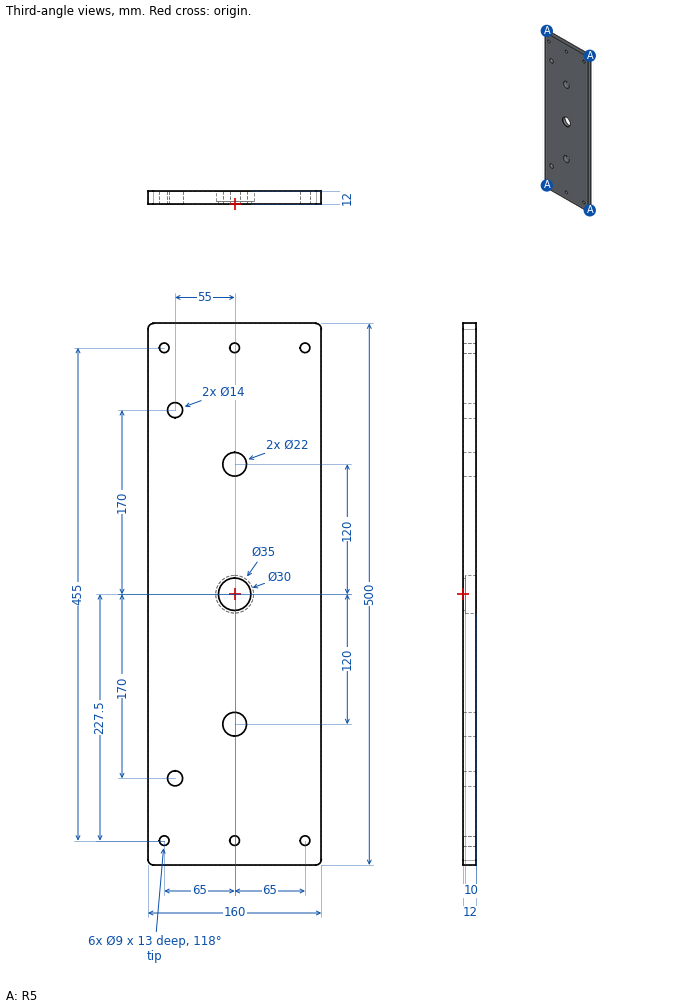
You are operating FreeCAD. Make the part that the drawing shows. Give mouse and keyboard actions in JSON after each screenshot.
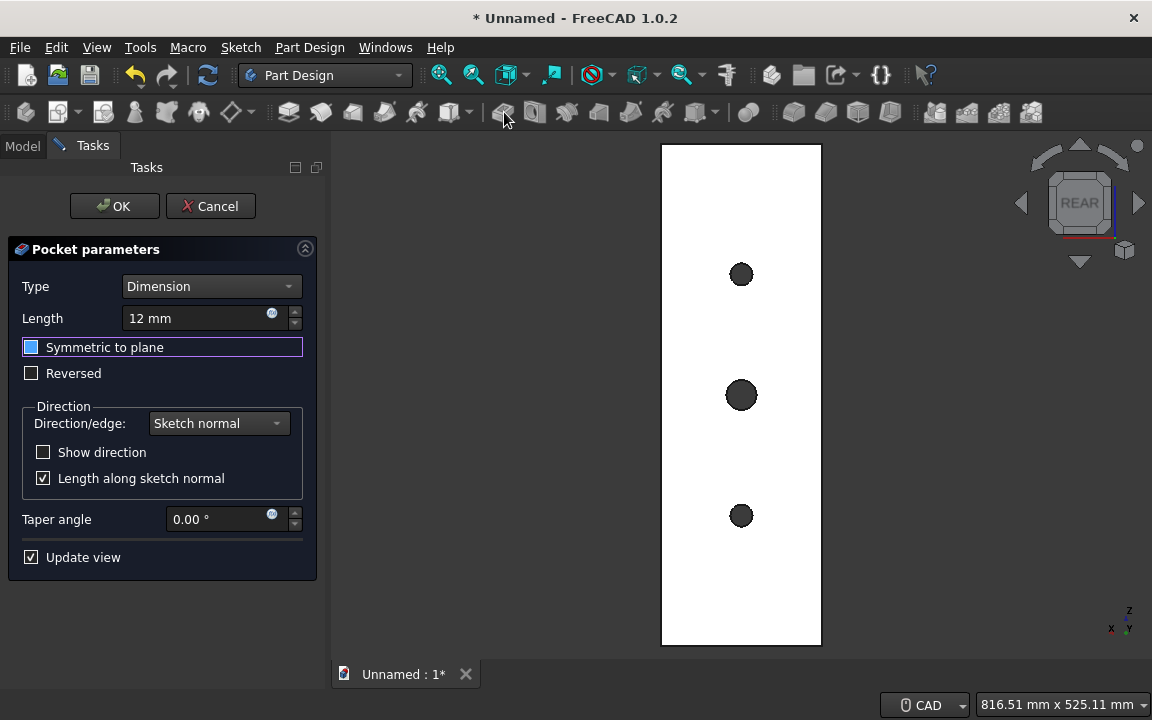
{"action": "left_click", "coordinate": [115, 206]}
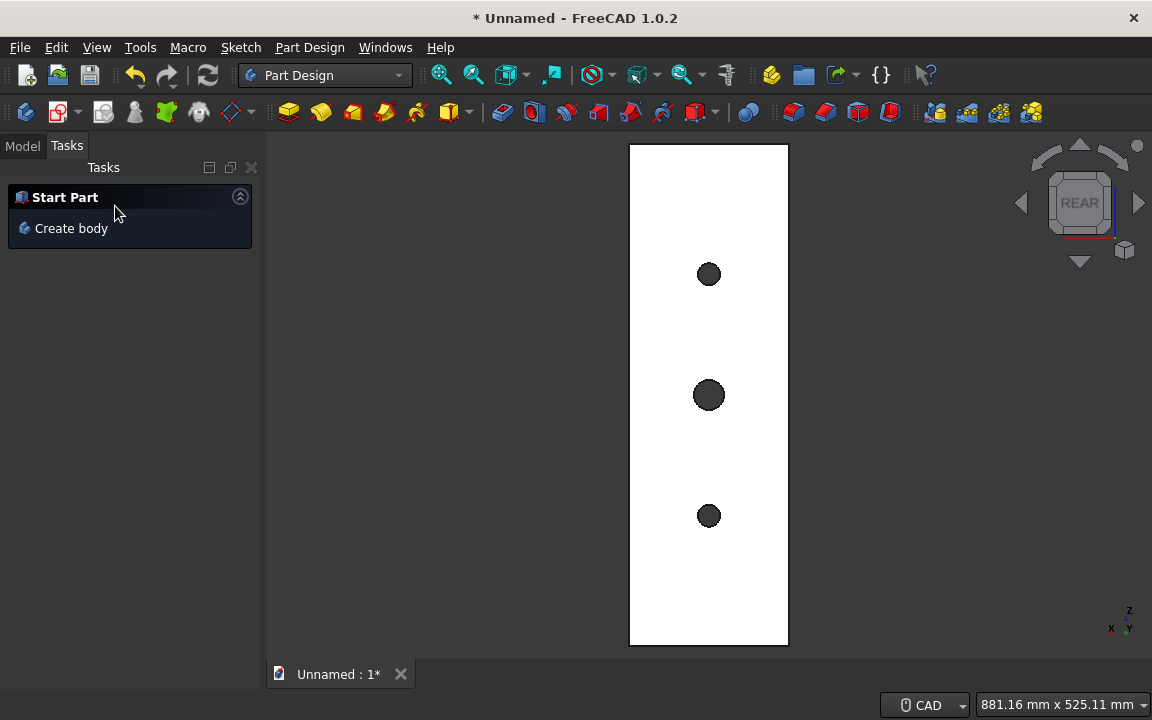
{"action": "left_click", "coordinate": [686, 466]}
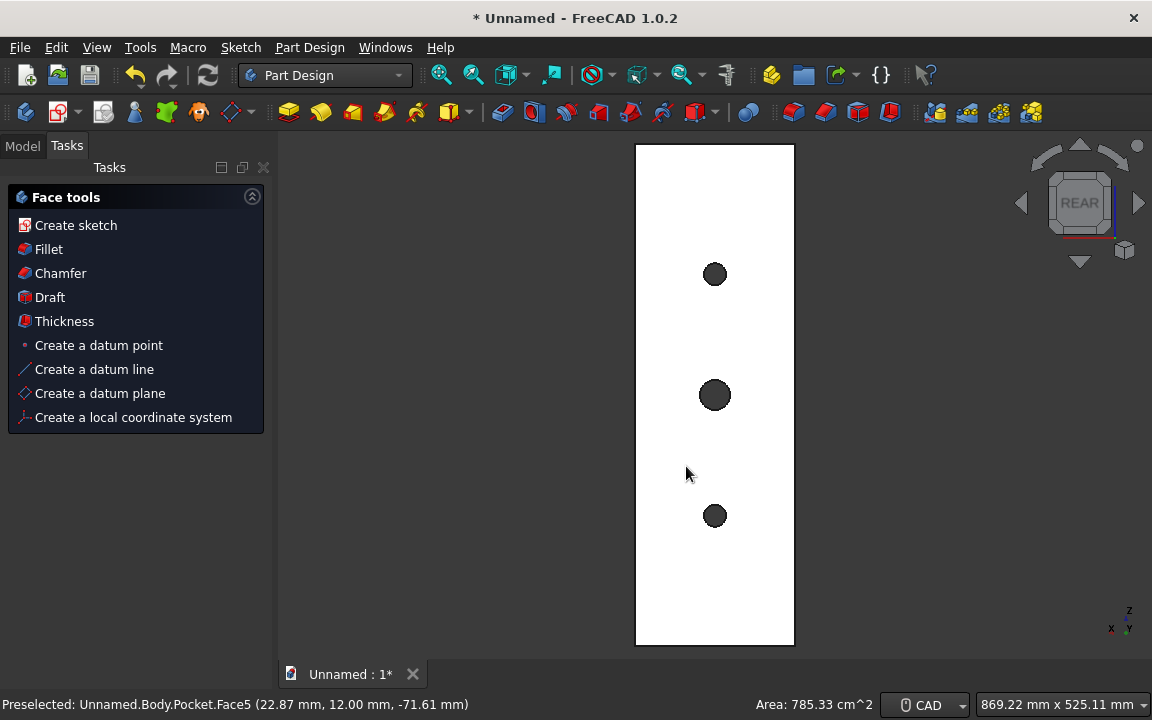
{"action": "left_click", "coordinate": [58, 112]}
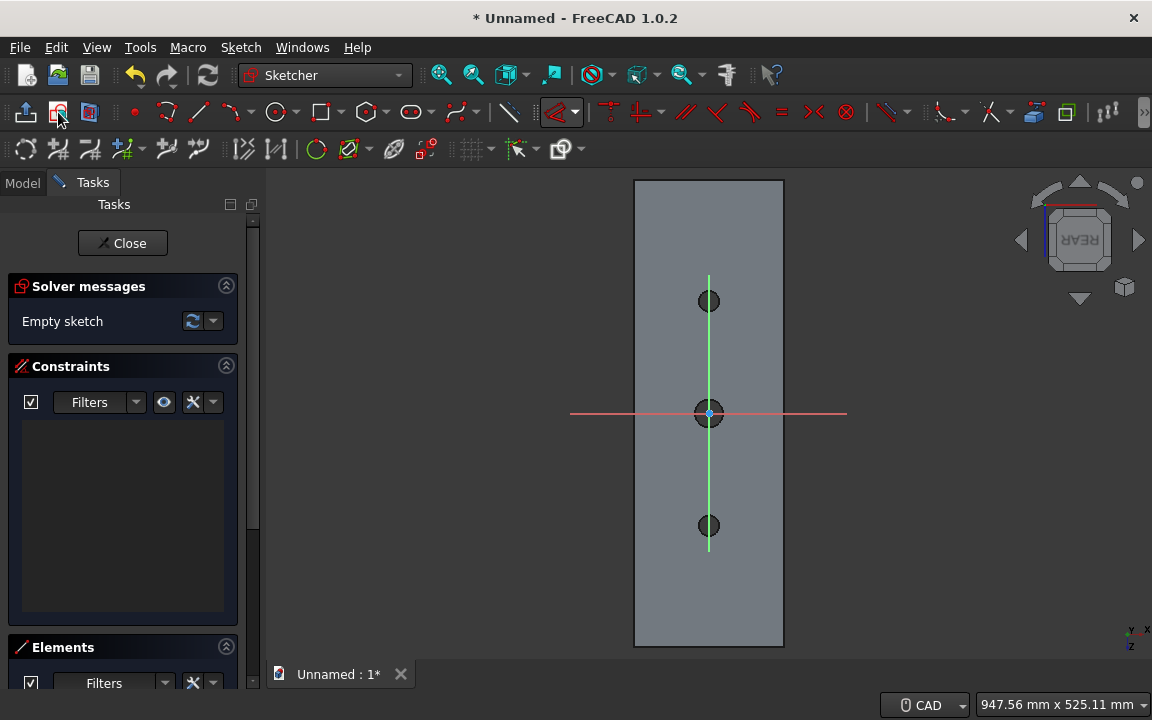
{"action": "scroll", "coordinate": [718, 413], "scroll_direction": "up", "scroll_amount": 11}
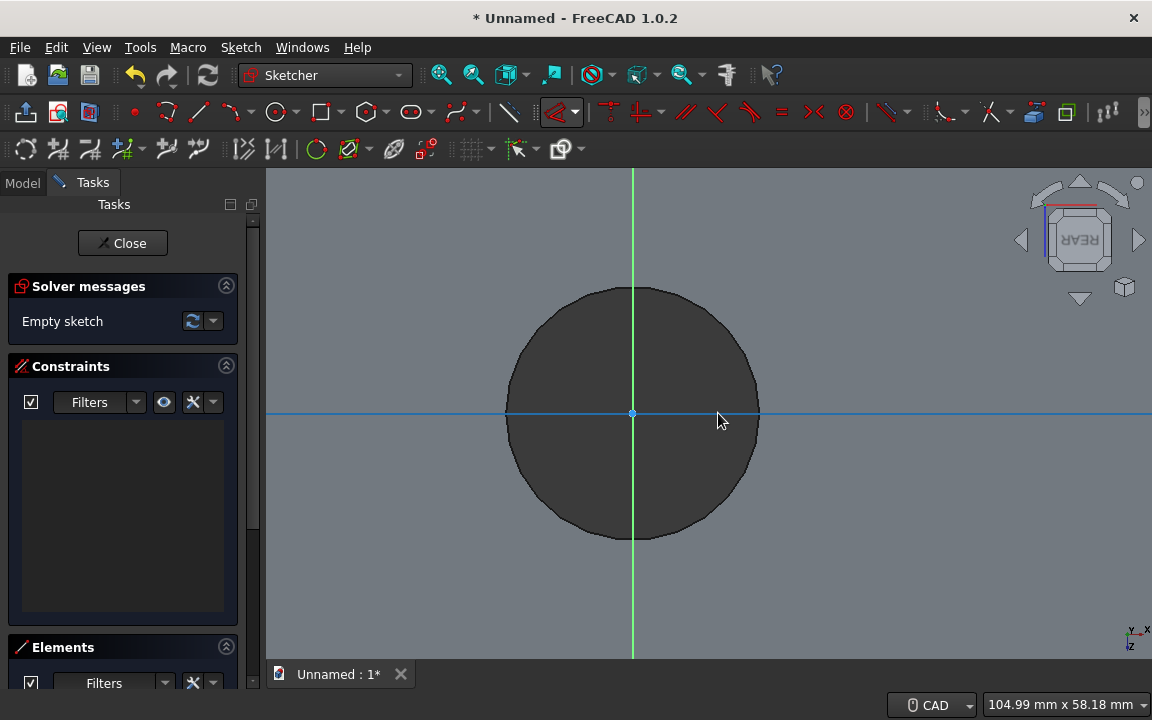
{"action": "key", "text": "g c"}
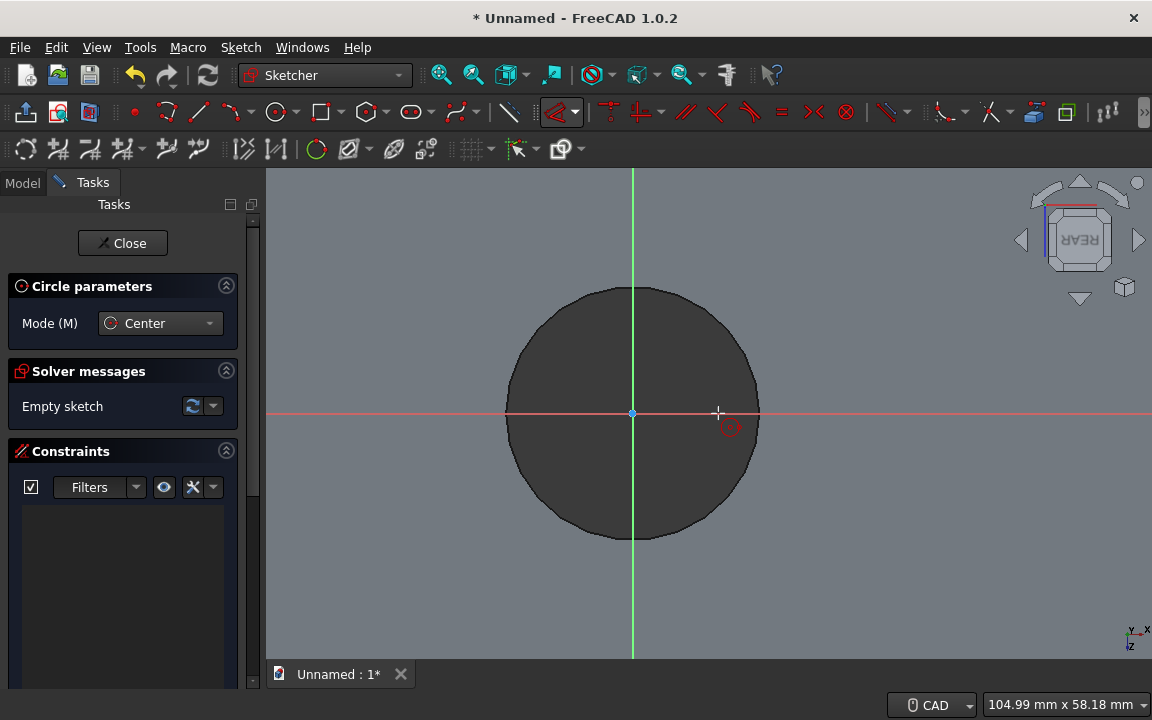
{"action": "left_click", "coordinate": [633, 413]}
{"action": "left_click", "coordinate": [737, 309]}
{"action": "key", "text": "Escape"}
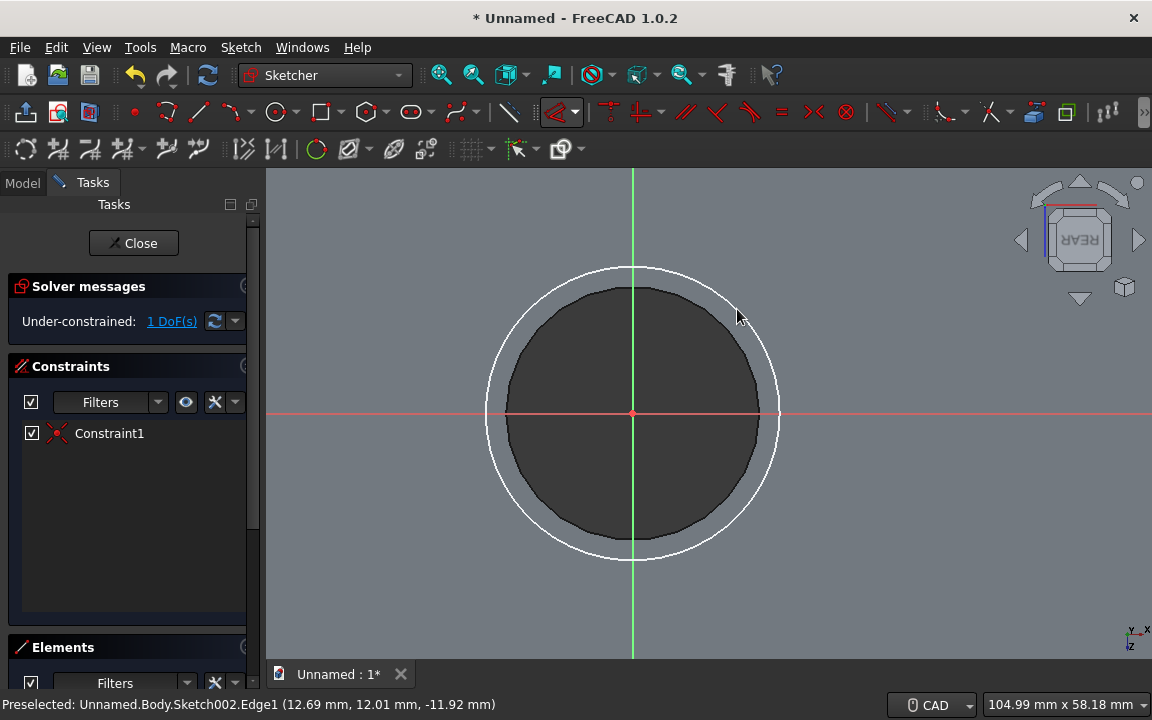
{"action": "left_click", "coordinate": [736, 309]}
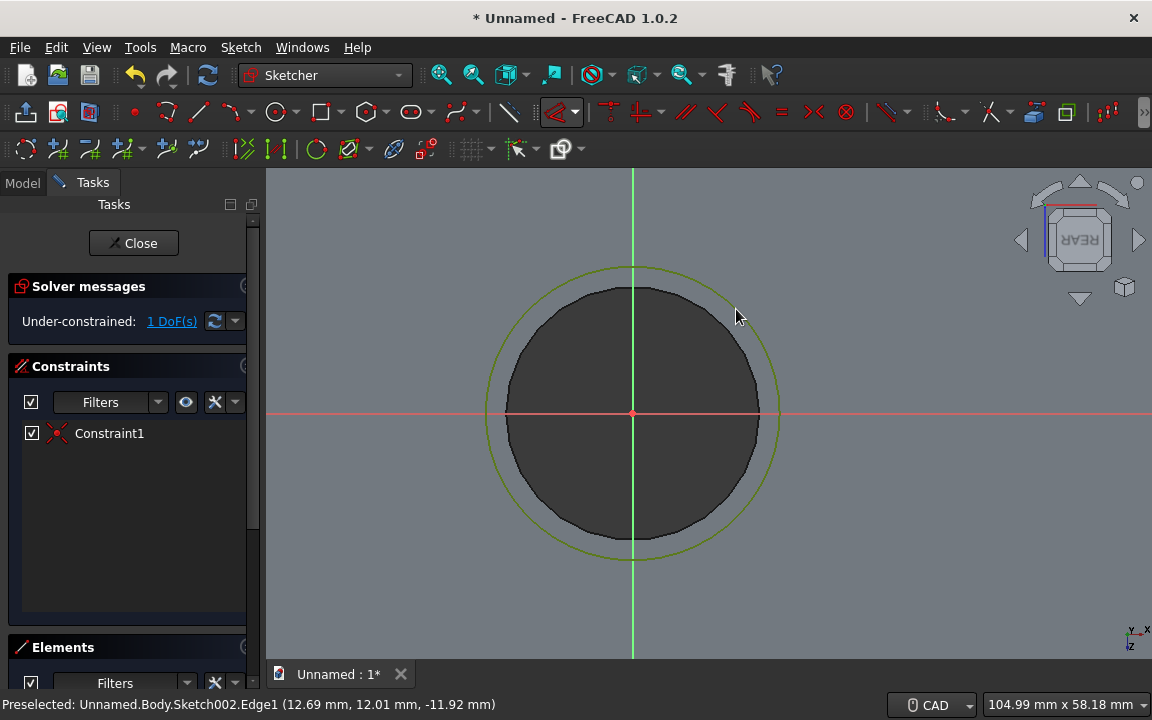
{"action": "key", "text": "k o"}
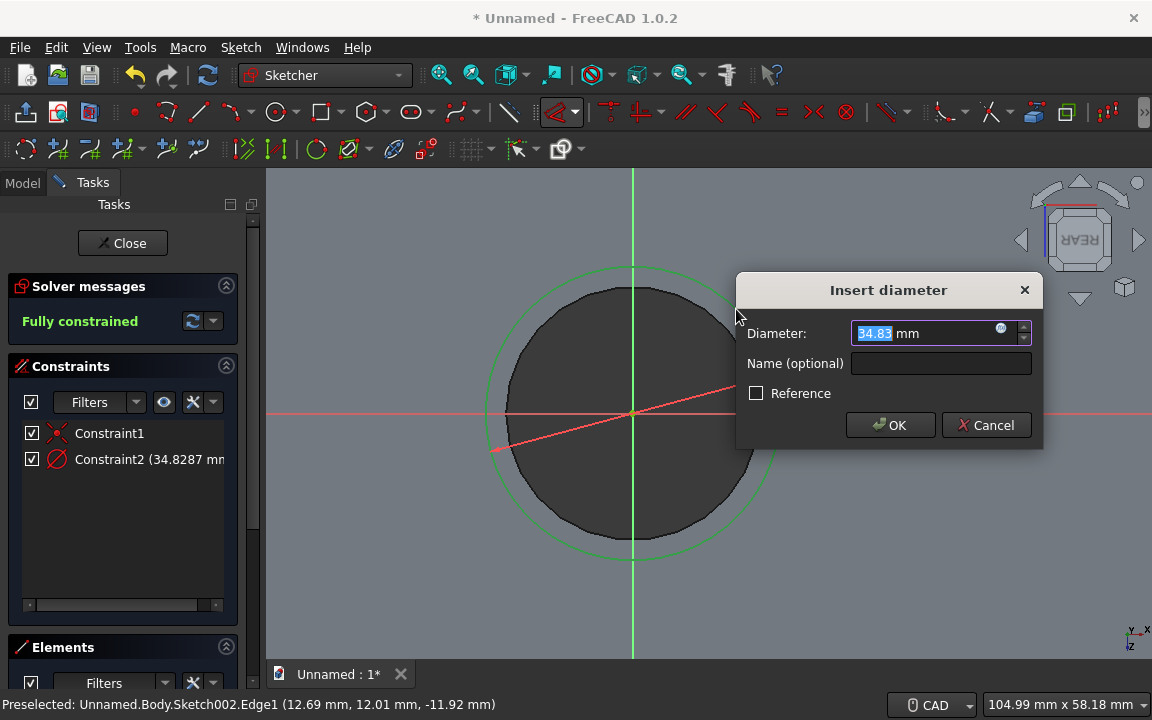
{"action": "type", "text": "35"}
{"action": "key", "text": "Return"}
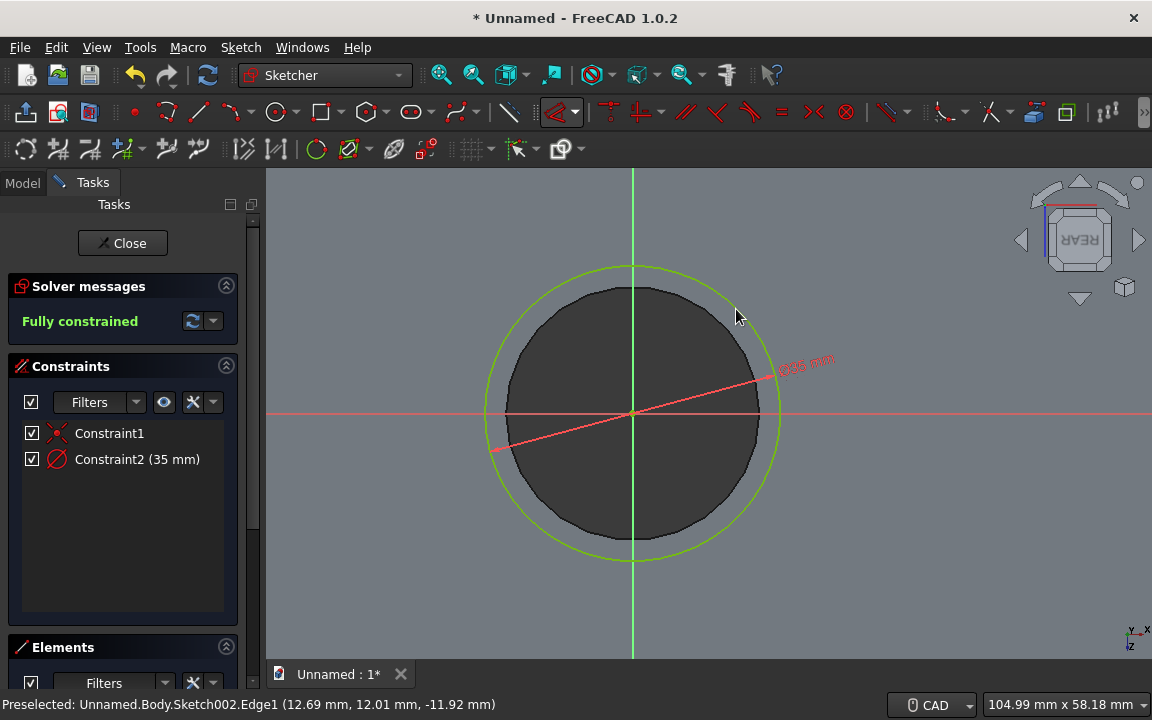
{"action": "left_click", "coordinate": [123, 243]}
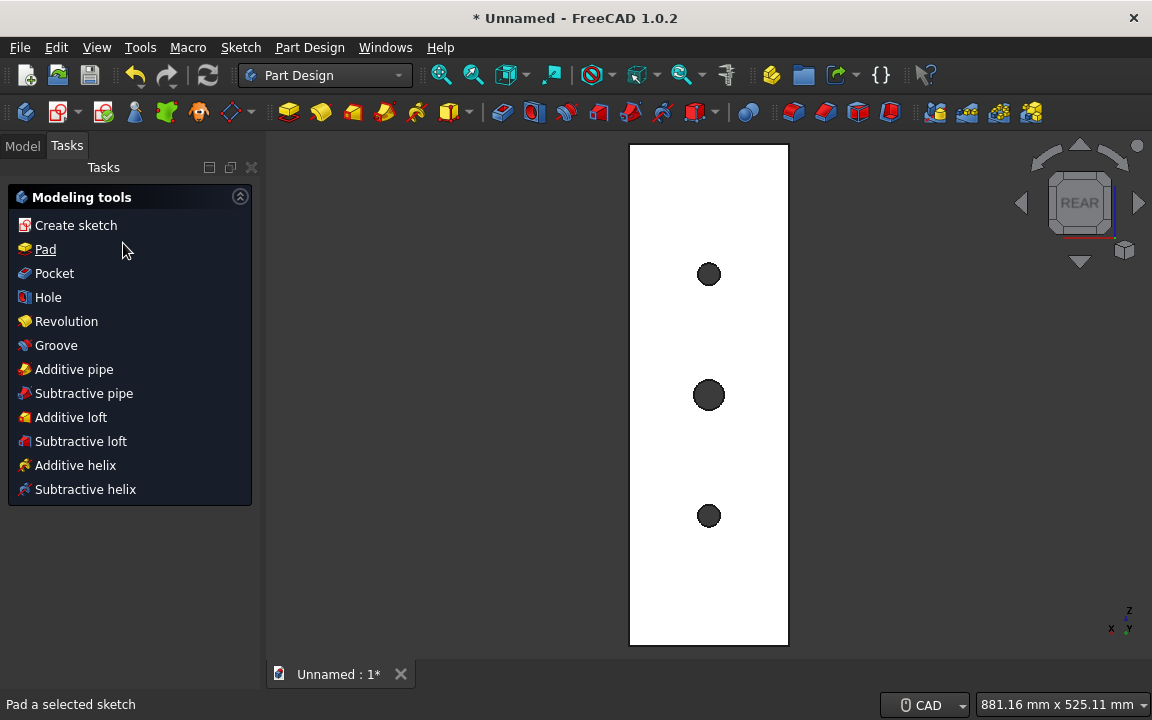
{"action": "left_click", "coordinate": [504, 112]}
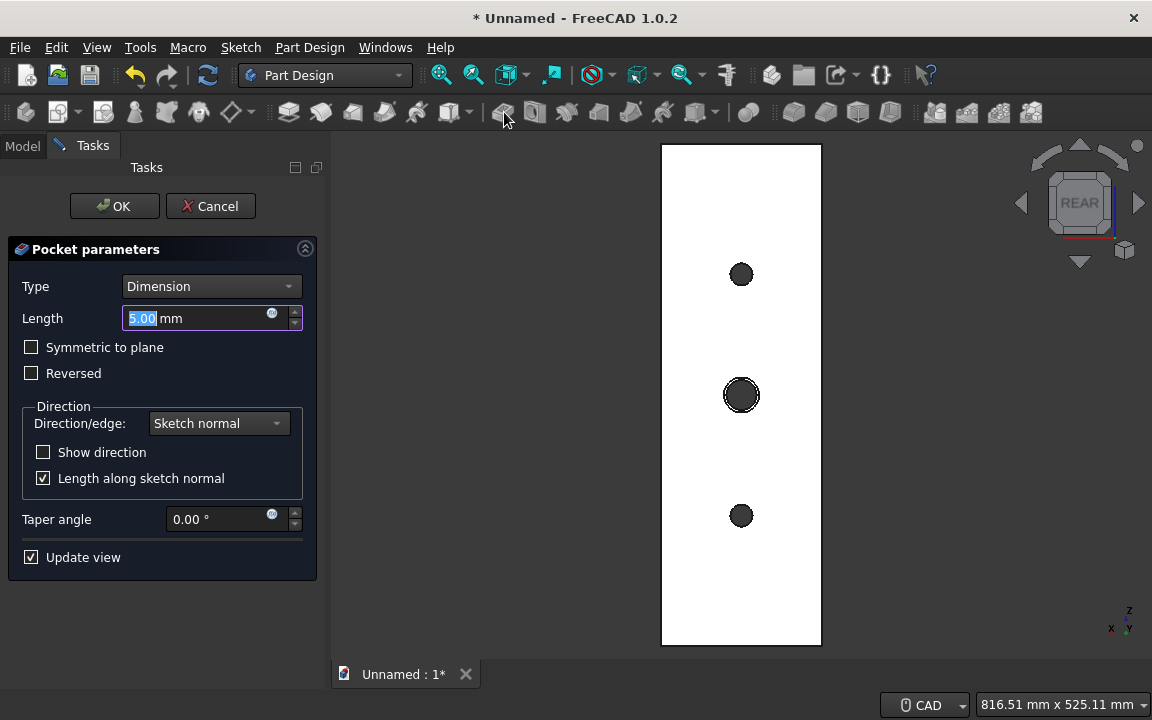
{"action": "type", "text": "10"}
{"action": "key", "text": "Tab"}